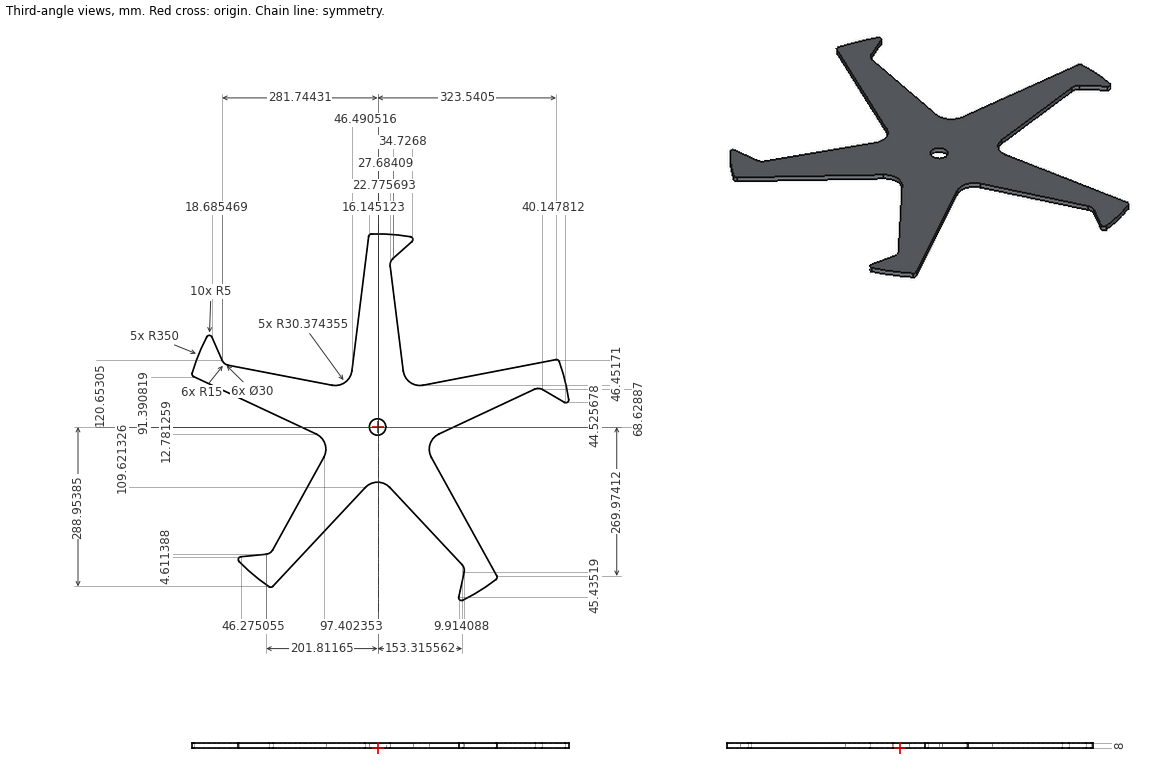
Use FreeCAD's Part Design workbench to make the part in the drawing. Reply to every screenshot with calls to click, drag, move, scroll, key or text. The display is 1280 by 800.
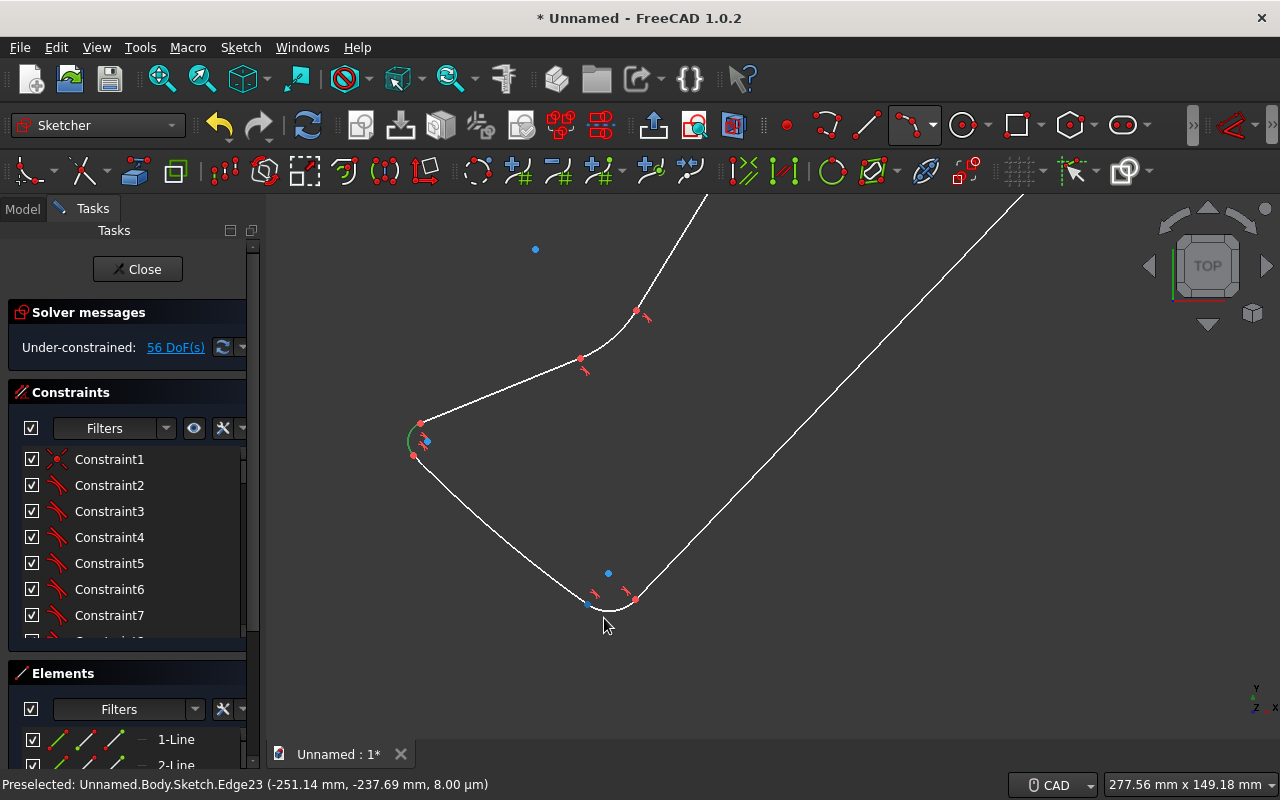
click(602, 610)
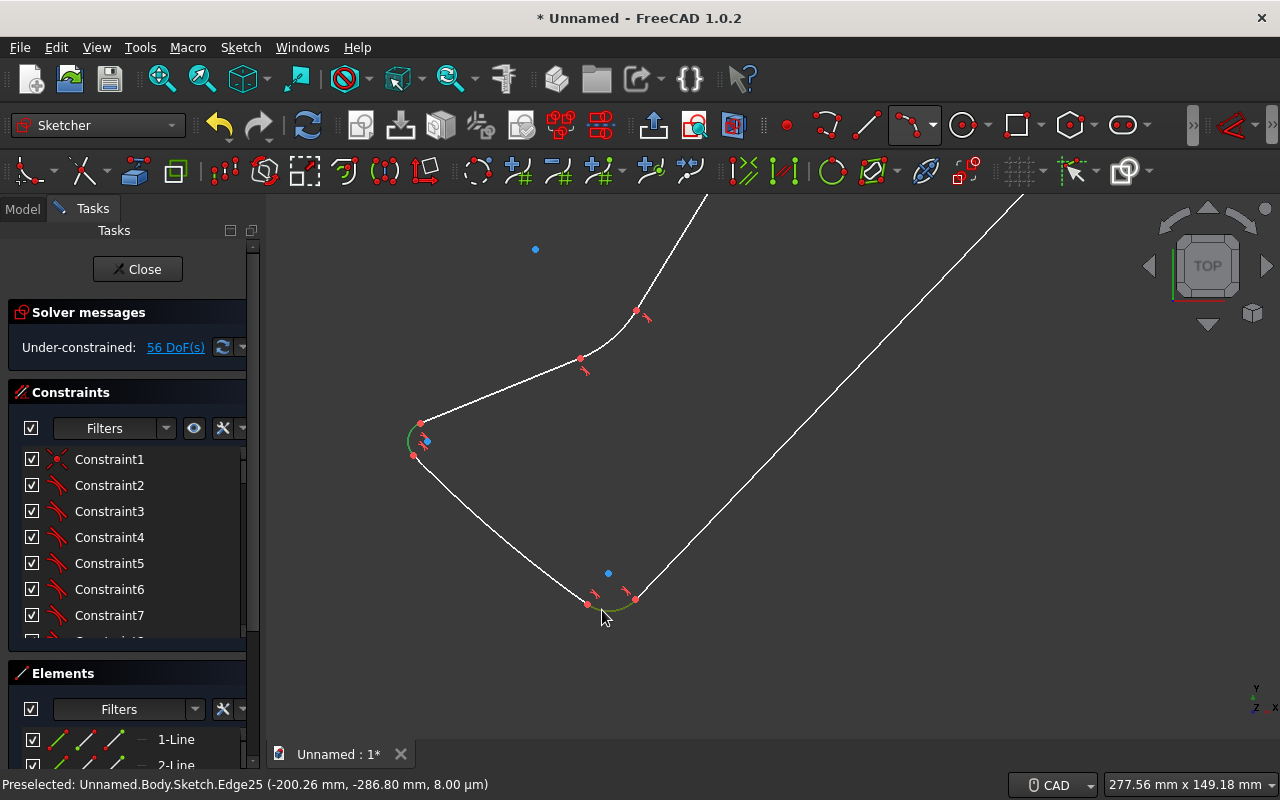
scroll(604, 618, down, 10)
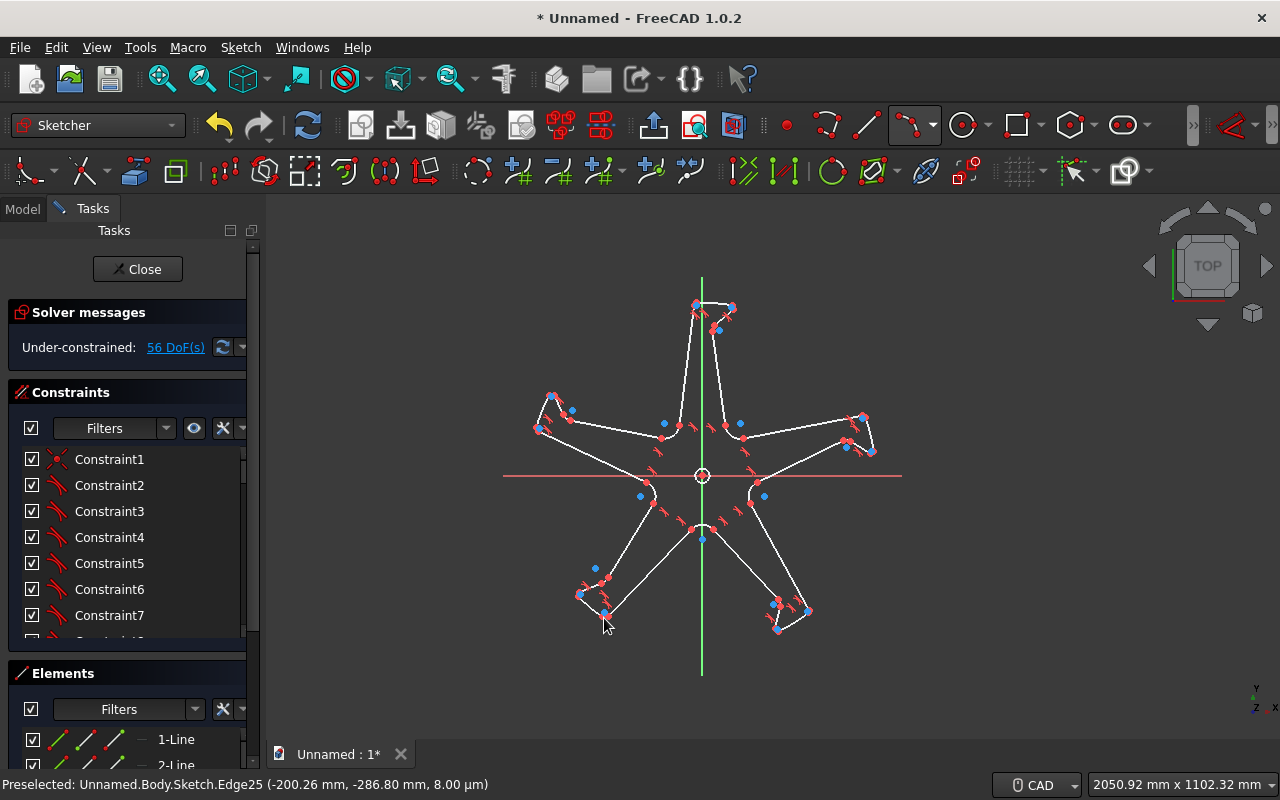
scroll(775, 630, up, 11)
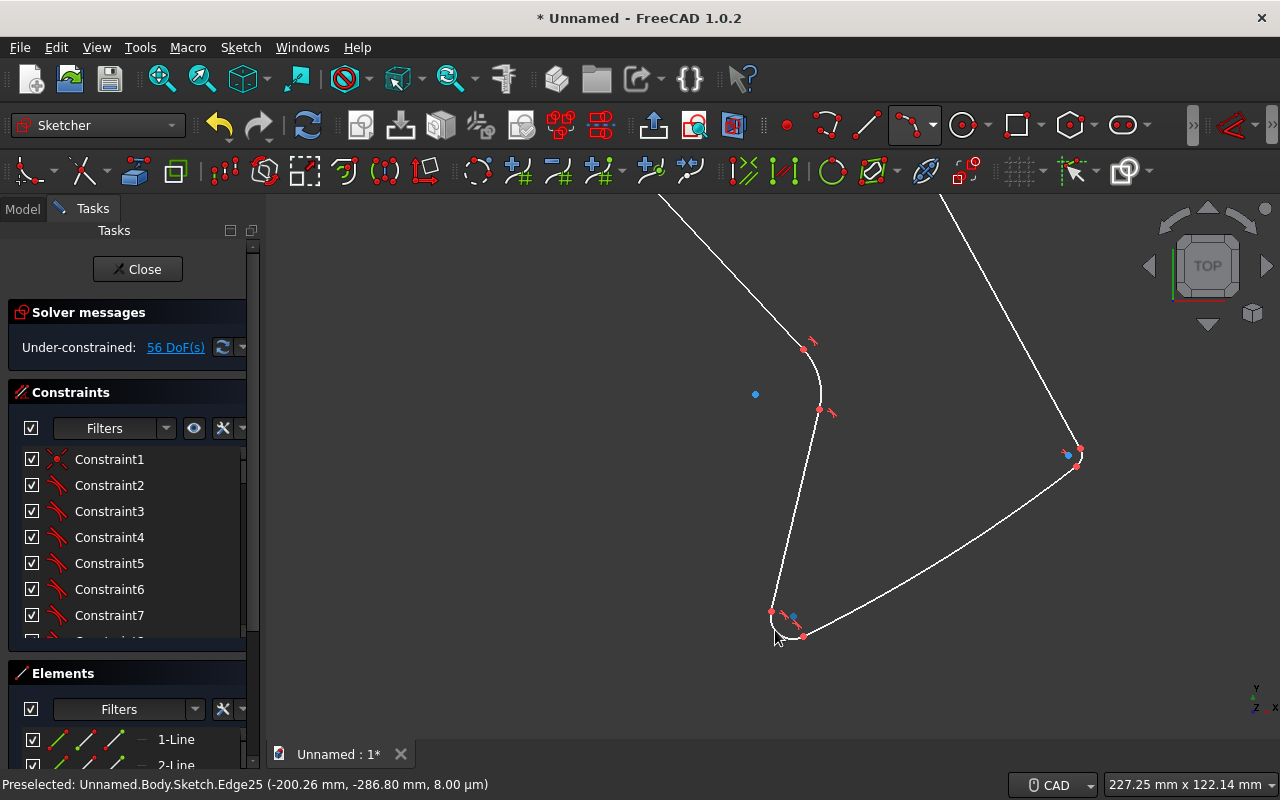
click(773, 626)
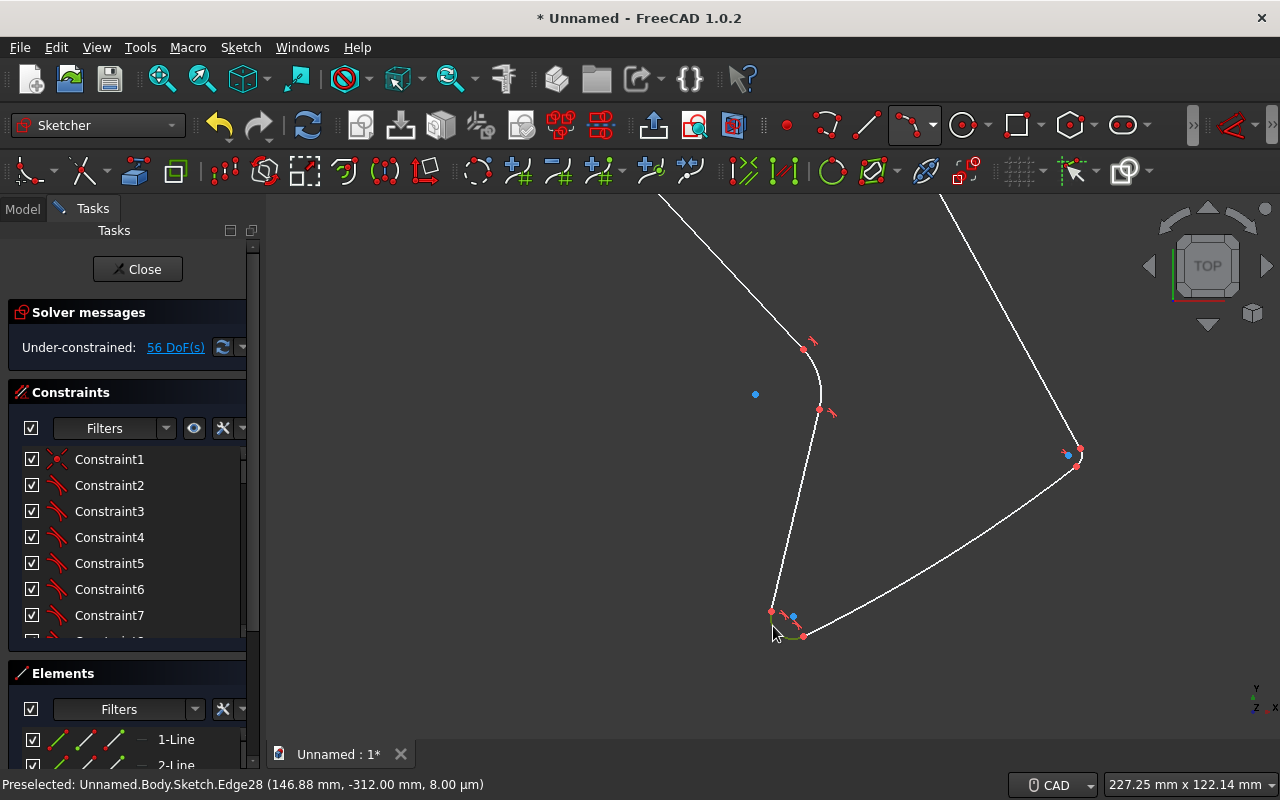
scroll(1082, 458, up, 2)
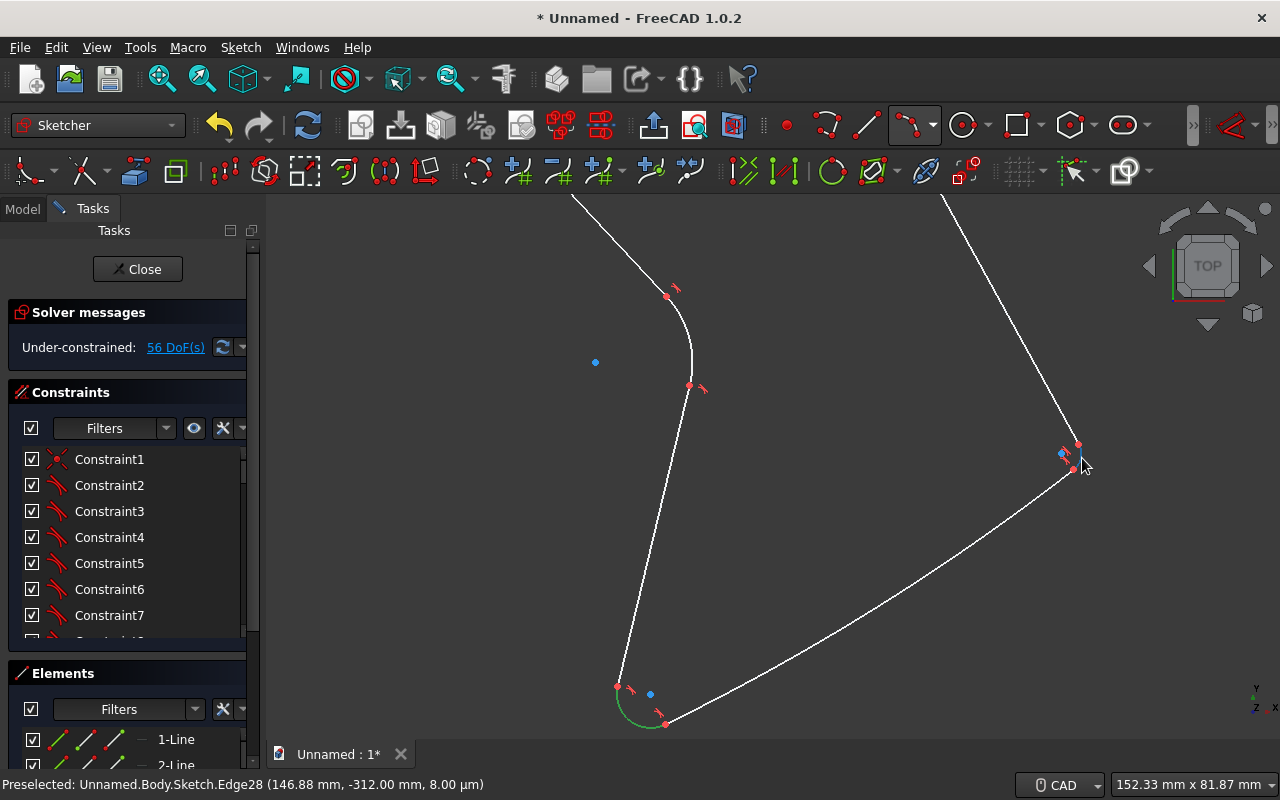
click(1081, 458)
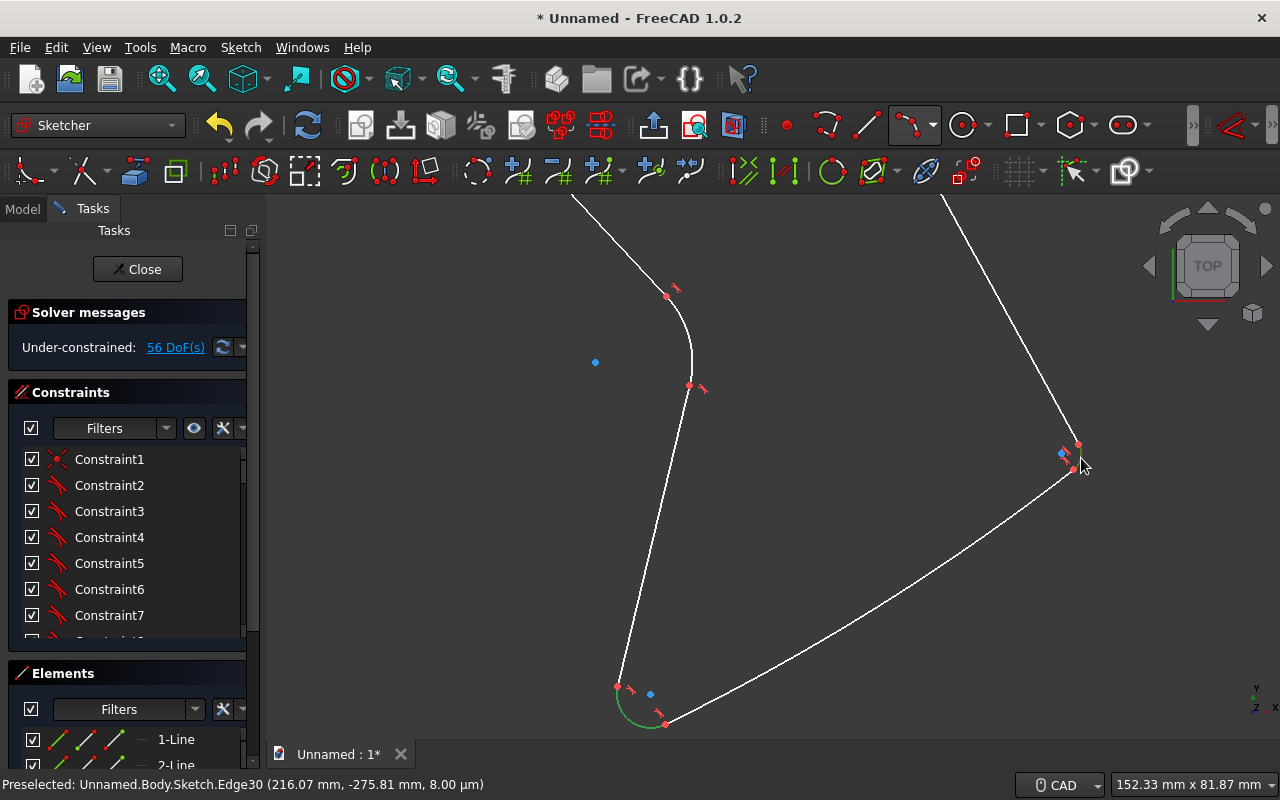
scroll(787, 624, down, 13)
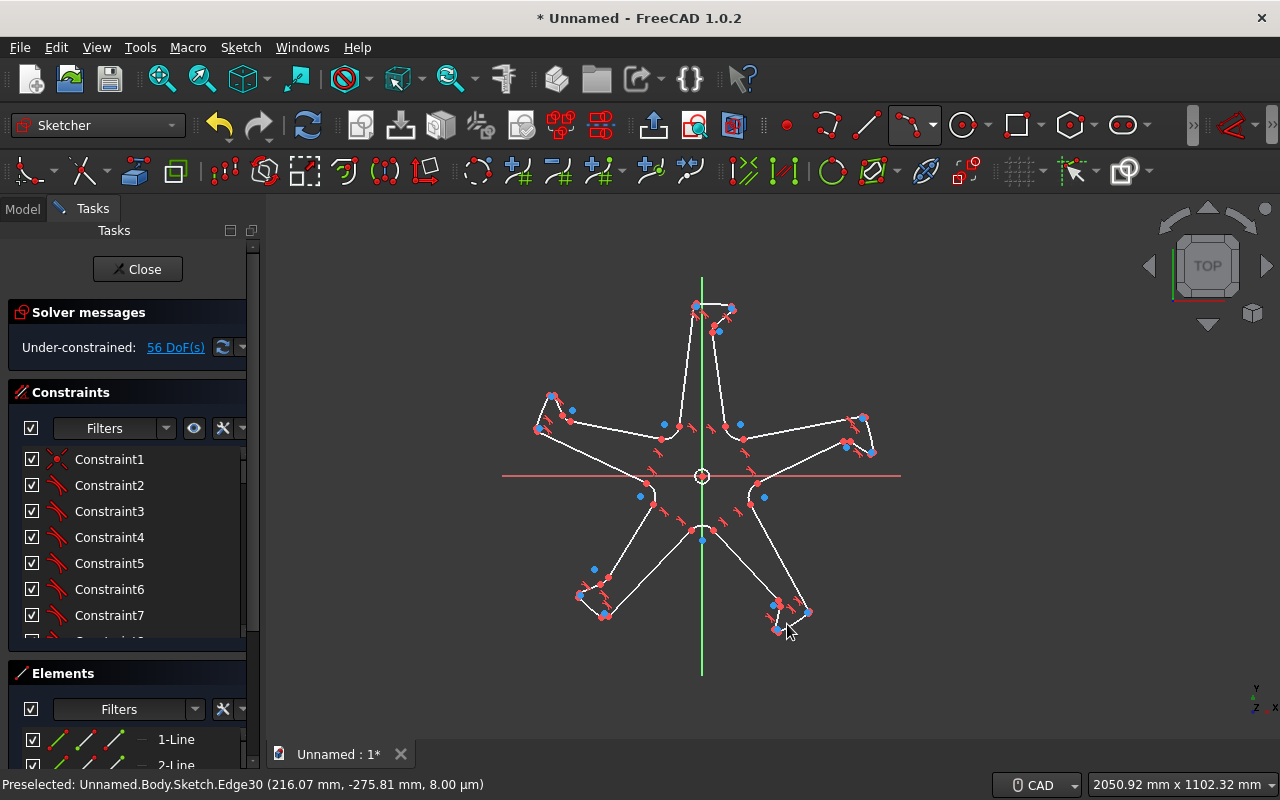
scroll(872, 455, up, 11)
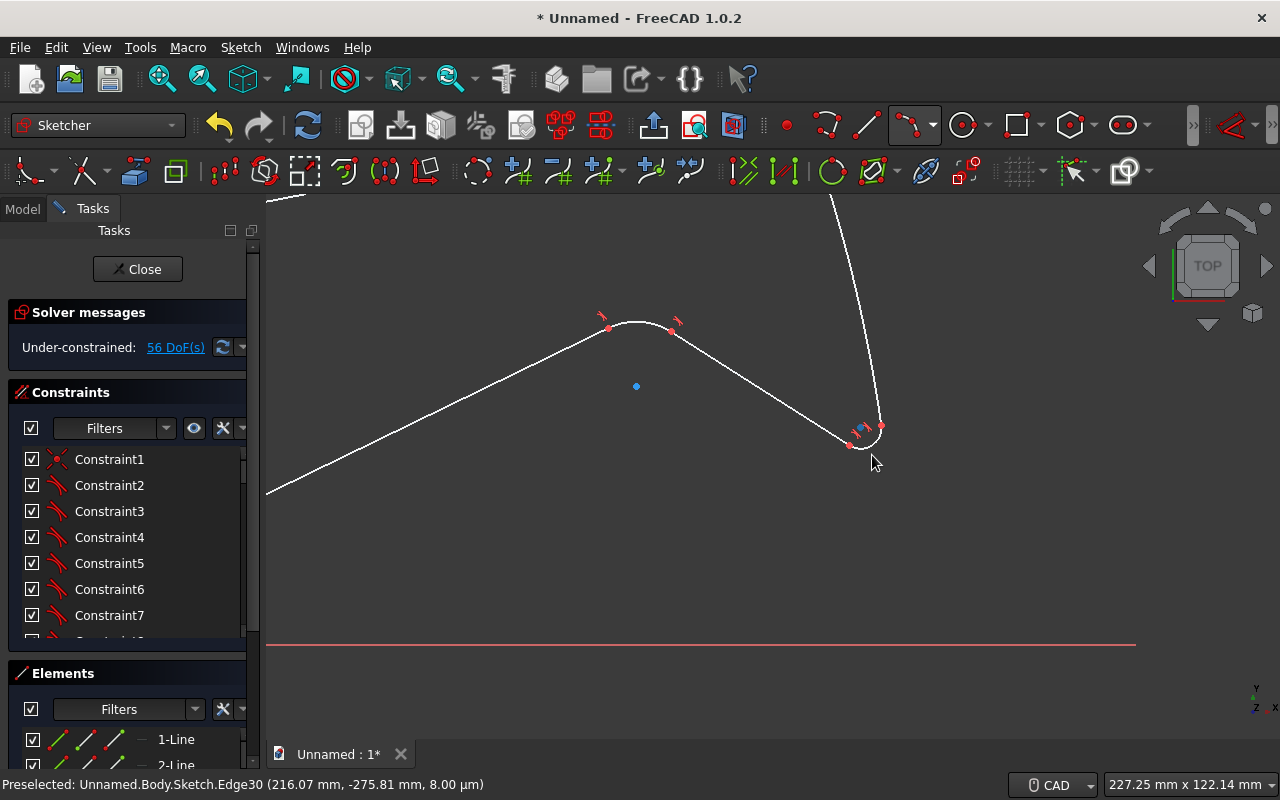
click(863, 449)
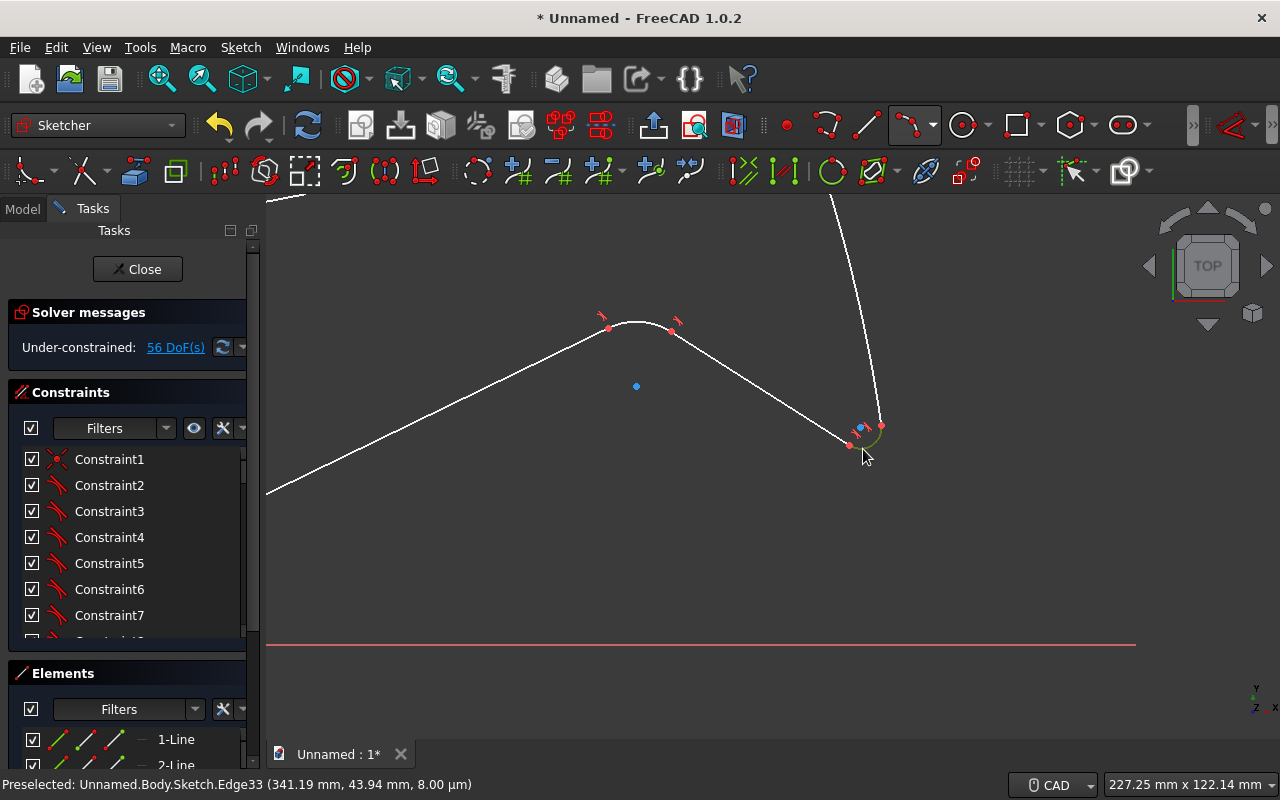
scroll(872, 454, down, 11)